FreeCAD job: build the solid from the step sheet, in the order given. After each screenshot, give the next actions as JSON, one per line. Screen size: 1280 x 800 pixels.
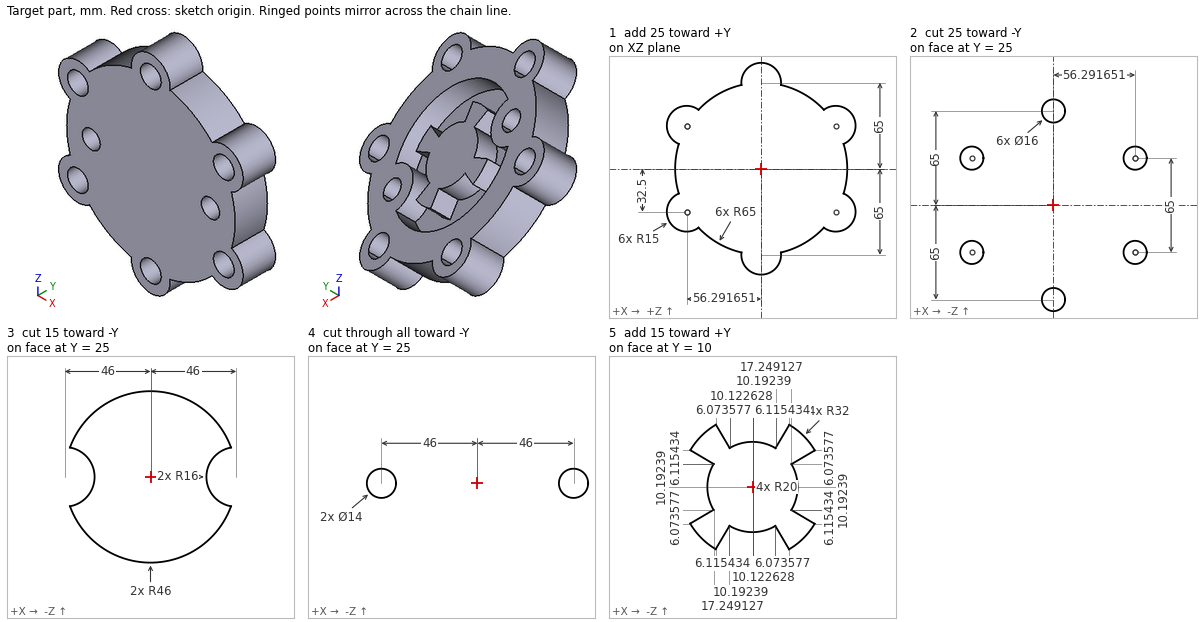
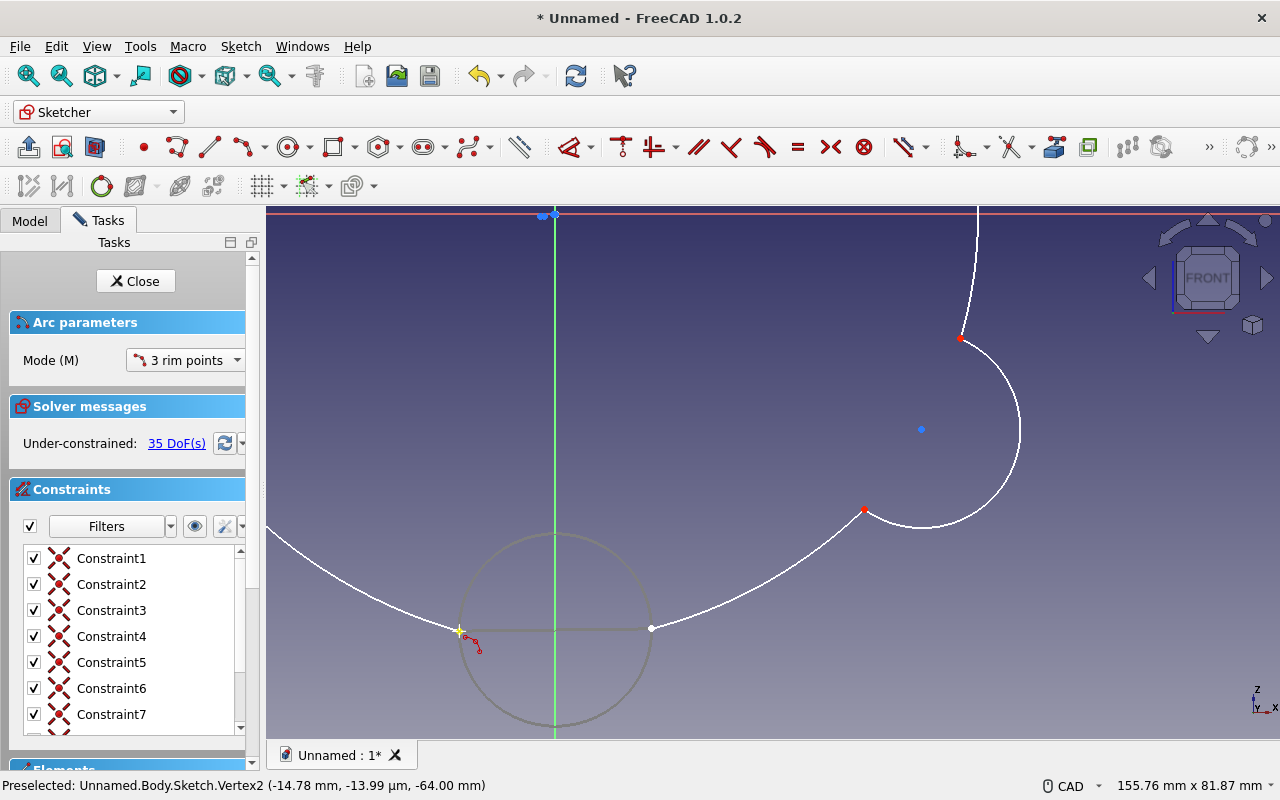
{"action": "scroll", "coordinate": [769, 584], "scroll_direction": "down", "scroll_amount": 6}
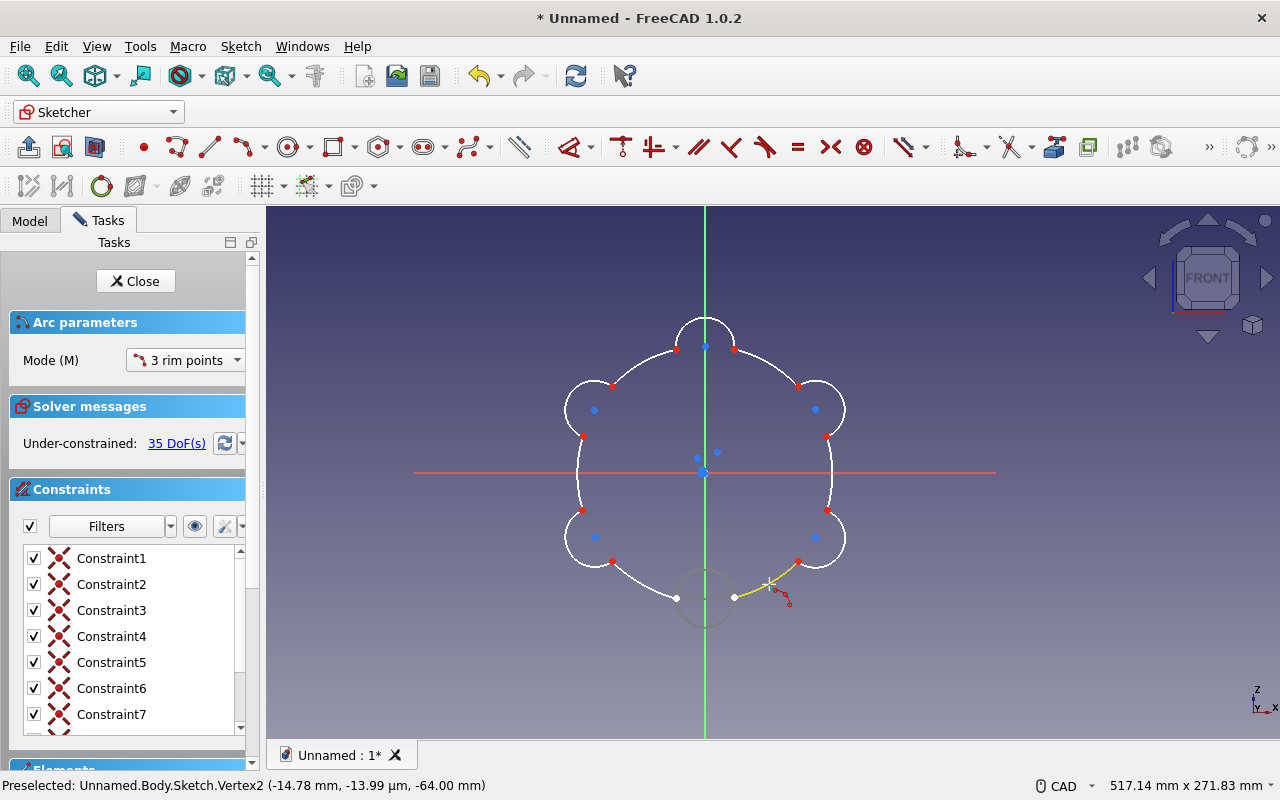
{"action": "left_click", "coordinate": [687, 624]}
{"action": "key", "text": "Escape"}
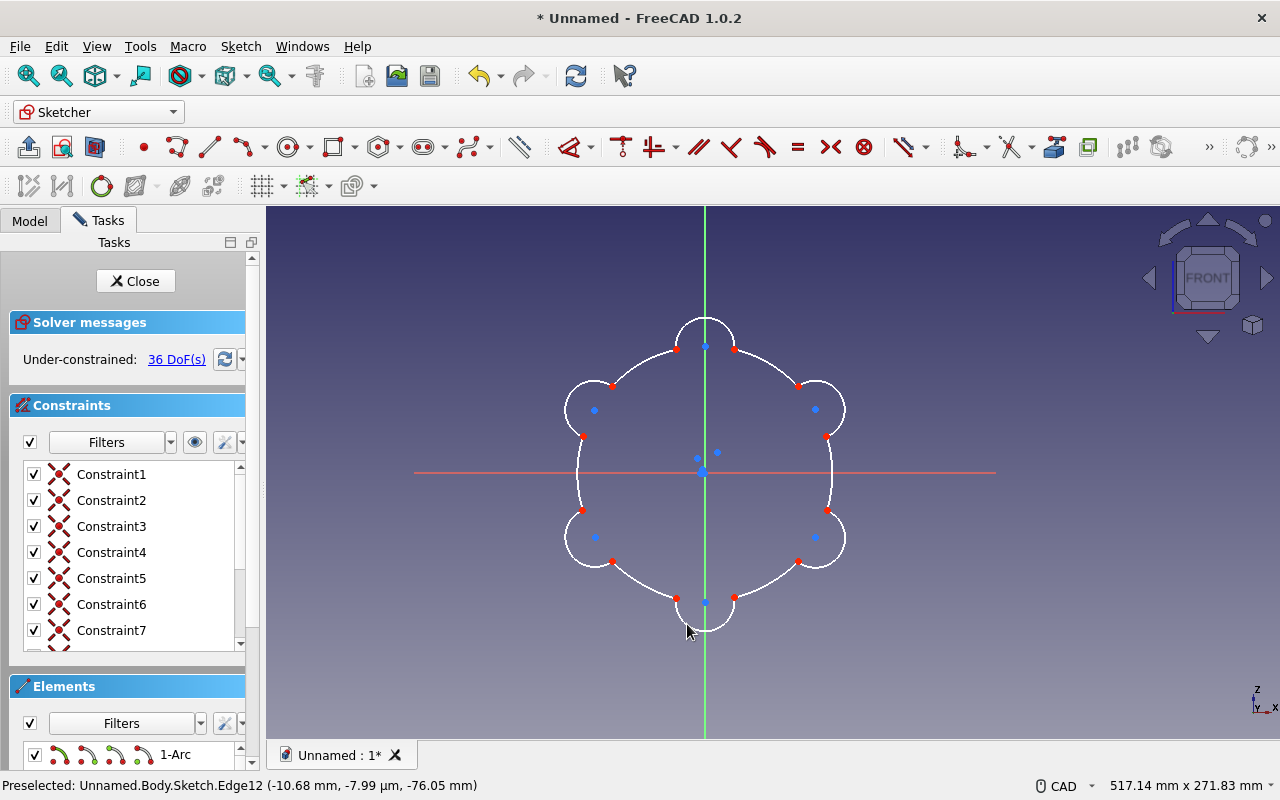
{"action": "left_click", "coordinate": [629, 576]}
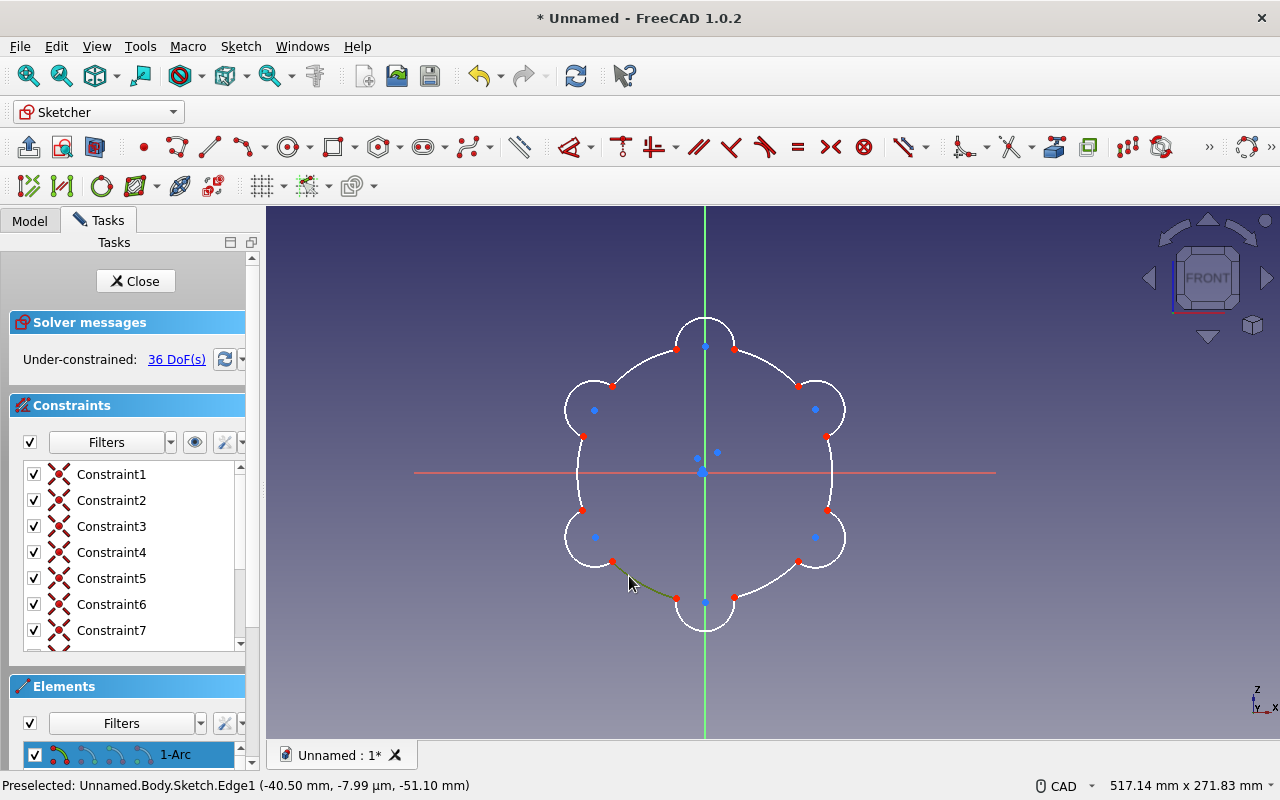
{"action": "left_click", "coordinate": [578, 459]}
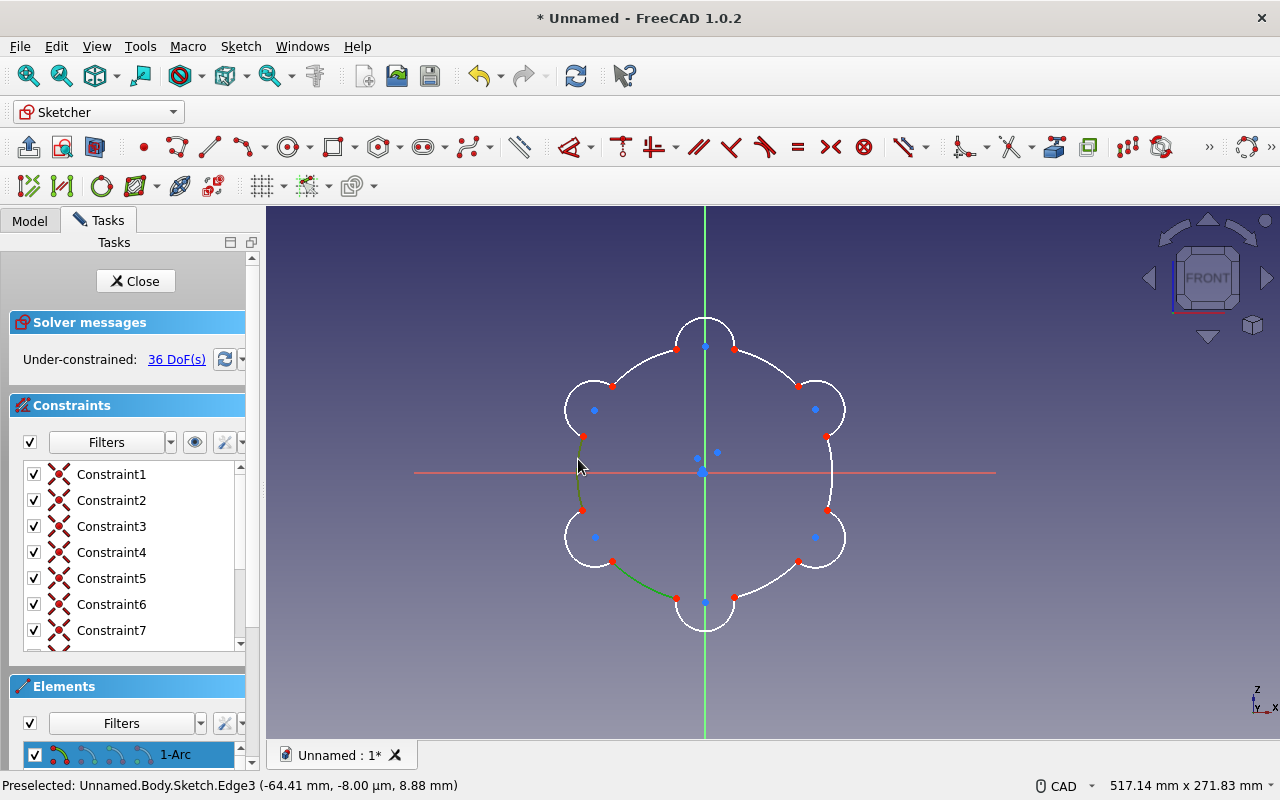
{"action": "left_click", "coordinate": [621, 148]}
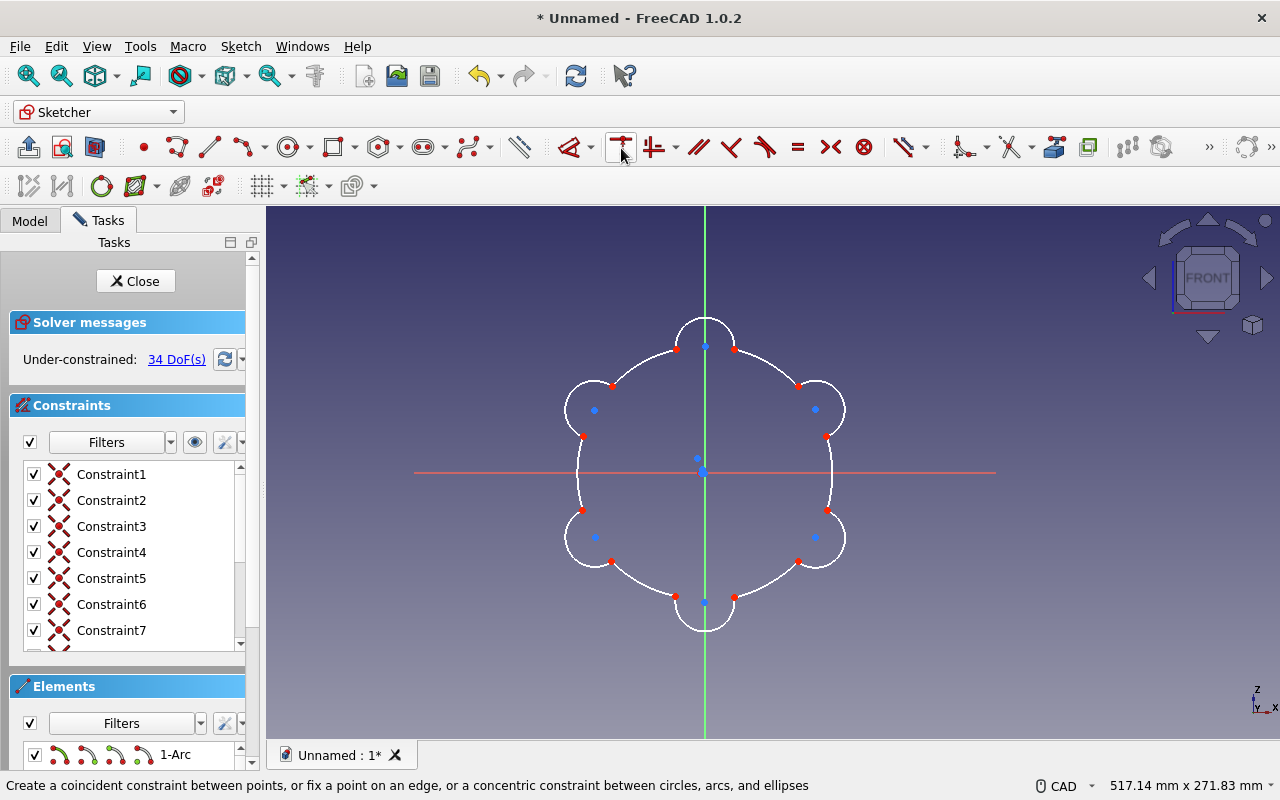
{"action": "left_click", "coordinate": [629, 576]}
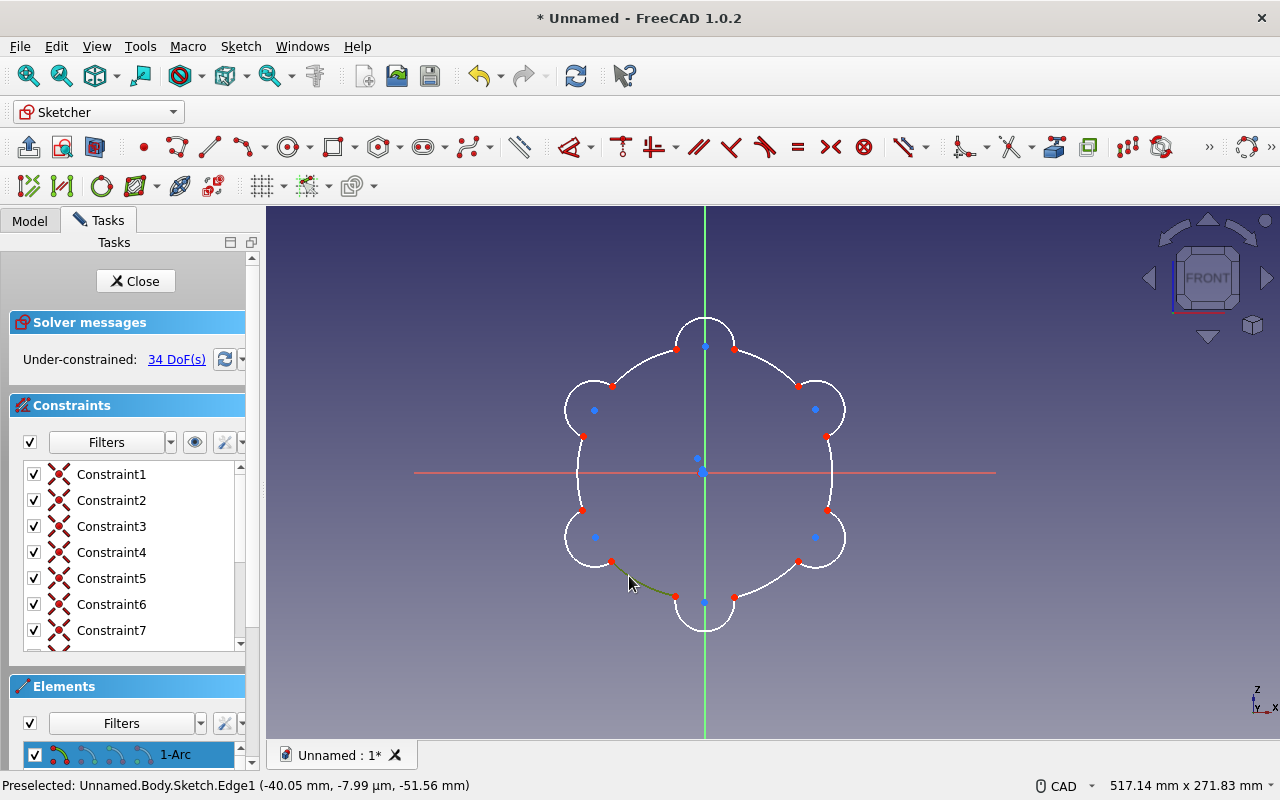
{"action": "left_click", "coordinate": [655, 357]}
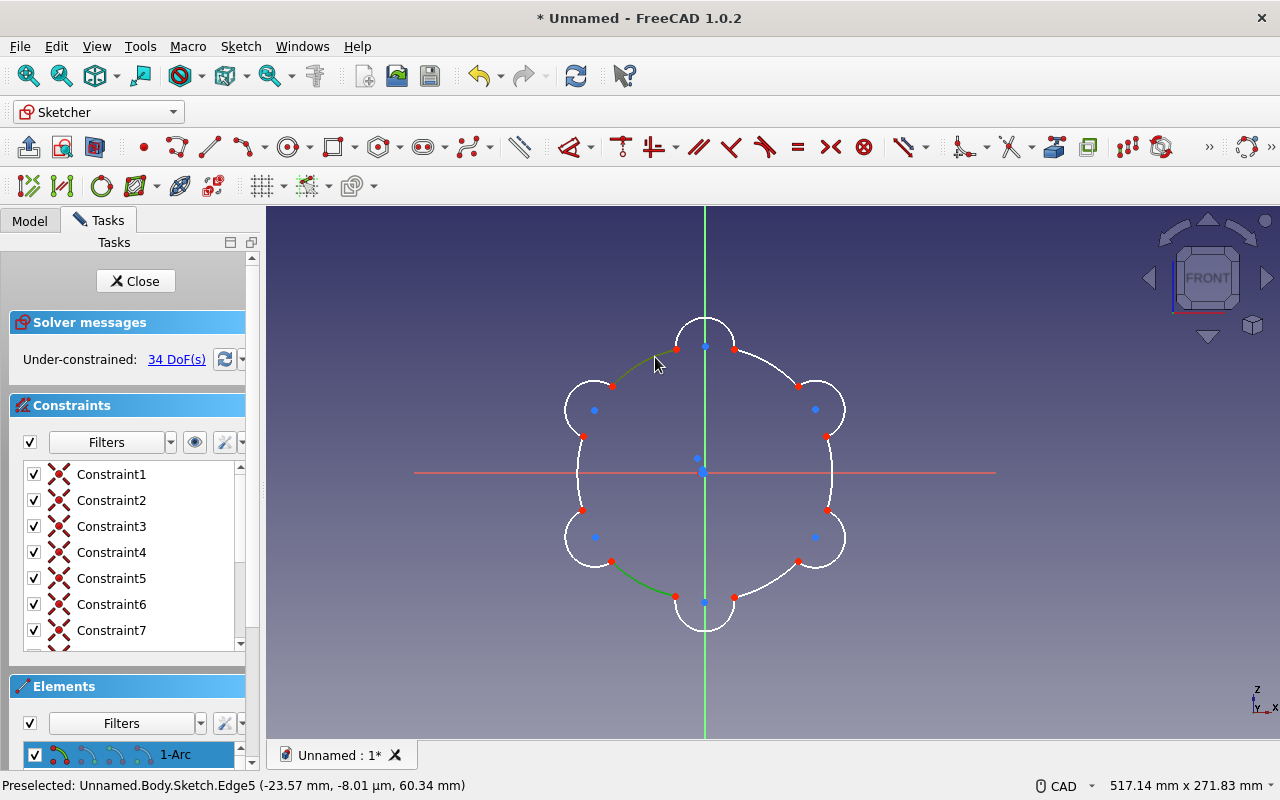
{"action": "left_click", "coordinate": [621, 148]}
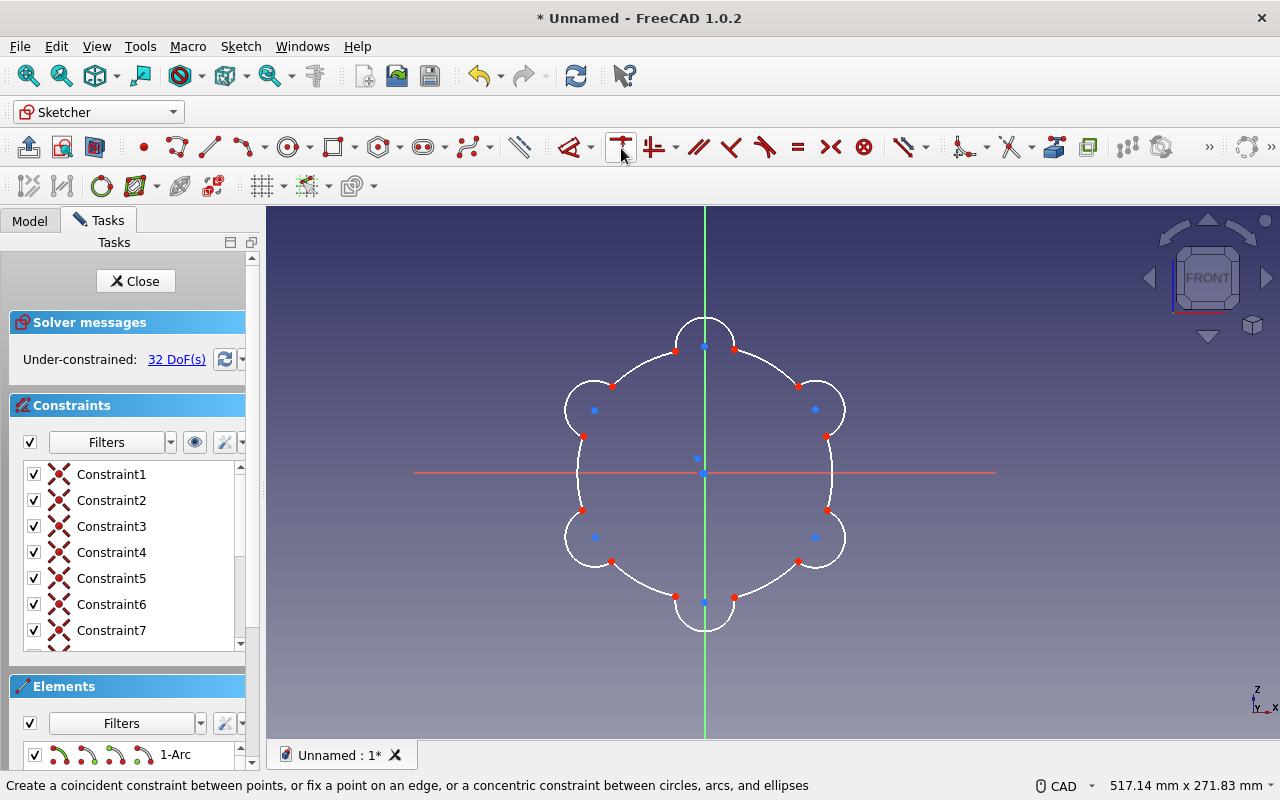
{"action": "left_click", "coordinate": [629, 576]}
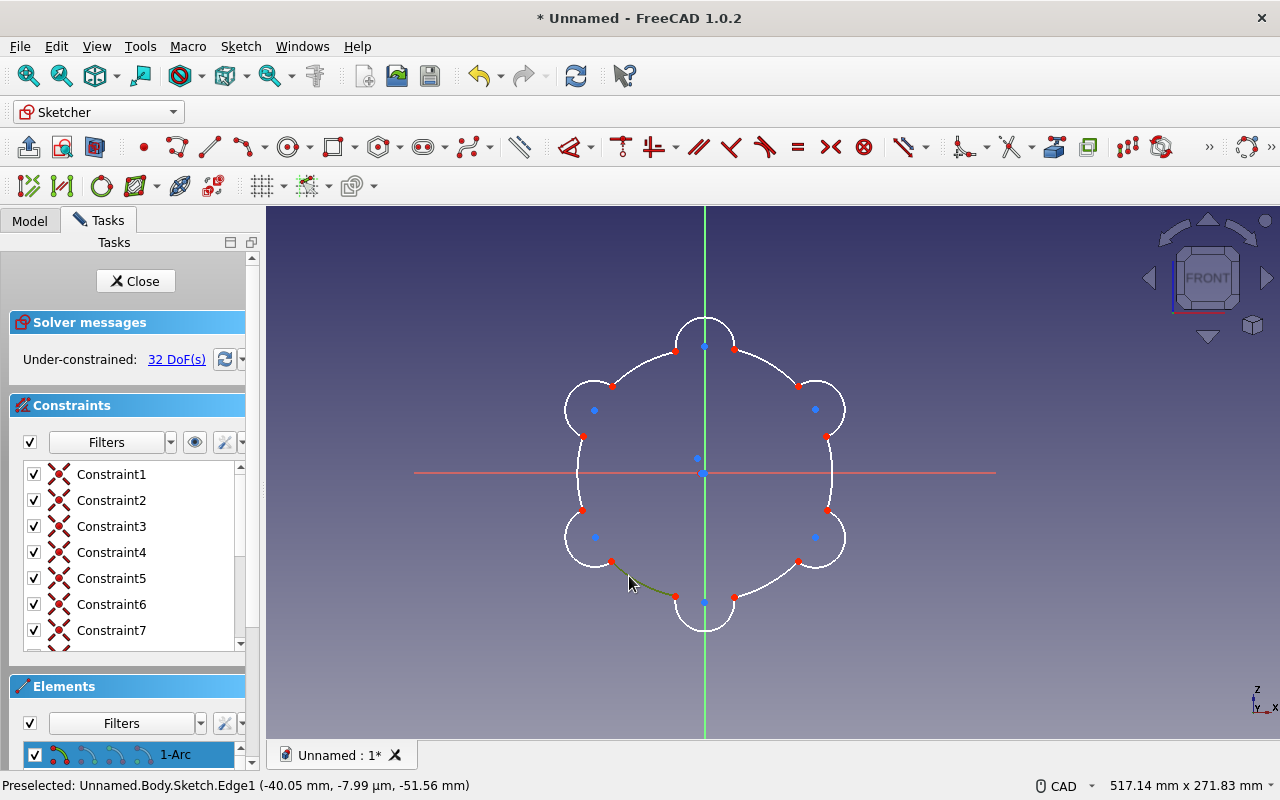
{"action": "left_click", "coordinate": [781, 372]}